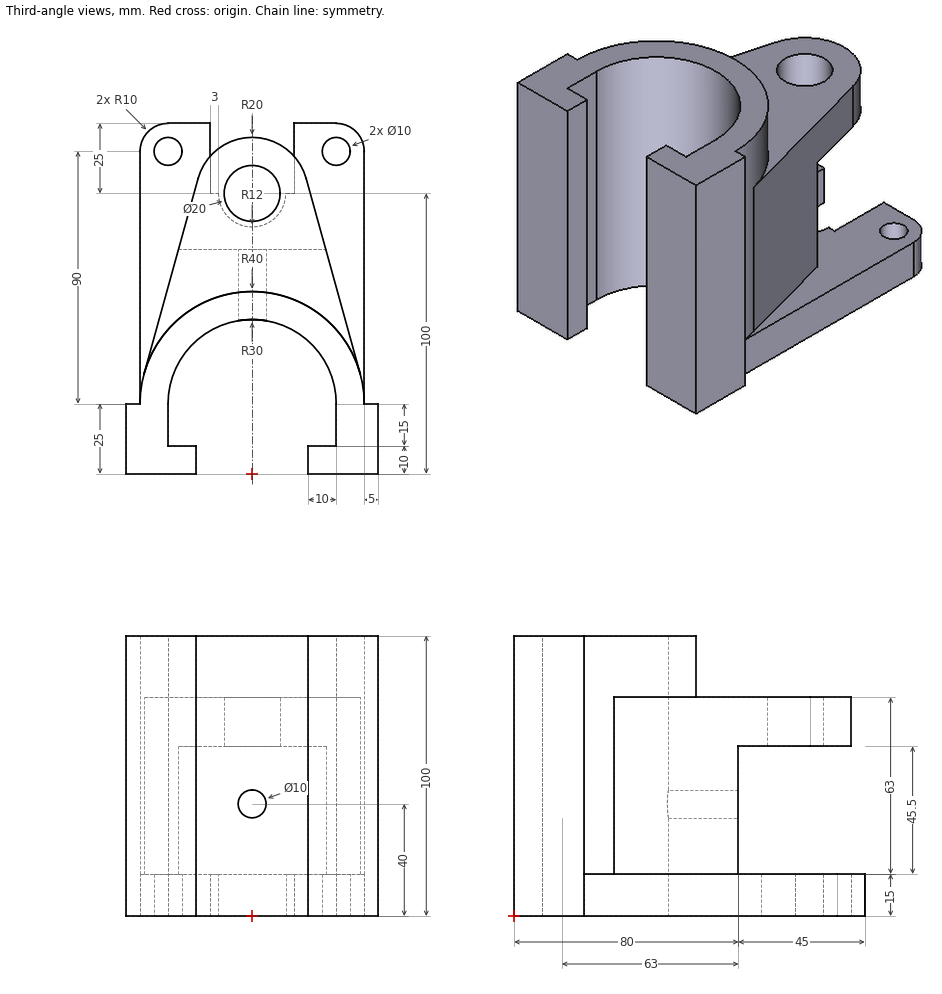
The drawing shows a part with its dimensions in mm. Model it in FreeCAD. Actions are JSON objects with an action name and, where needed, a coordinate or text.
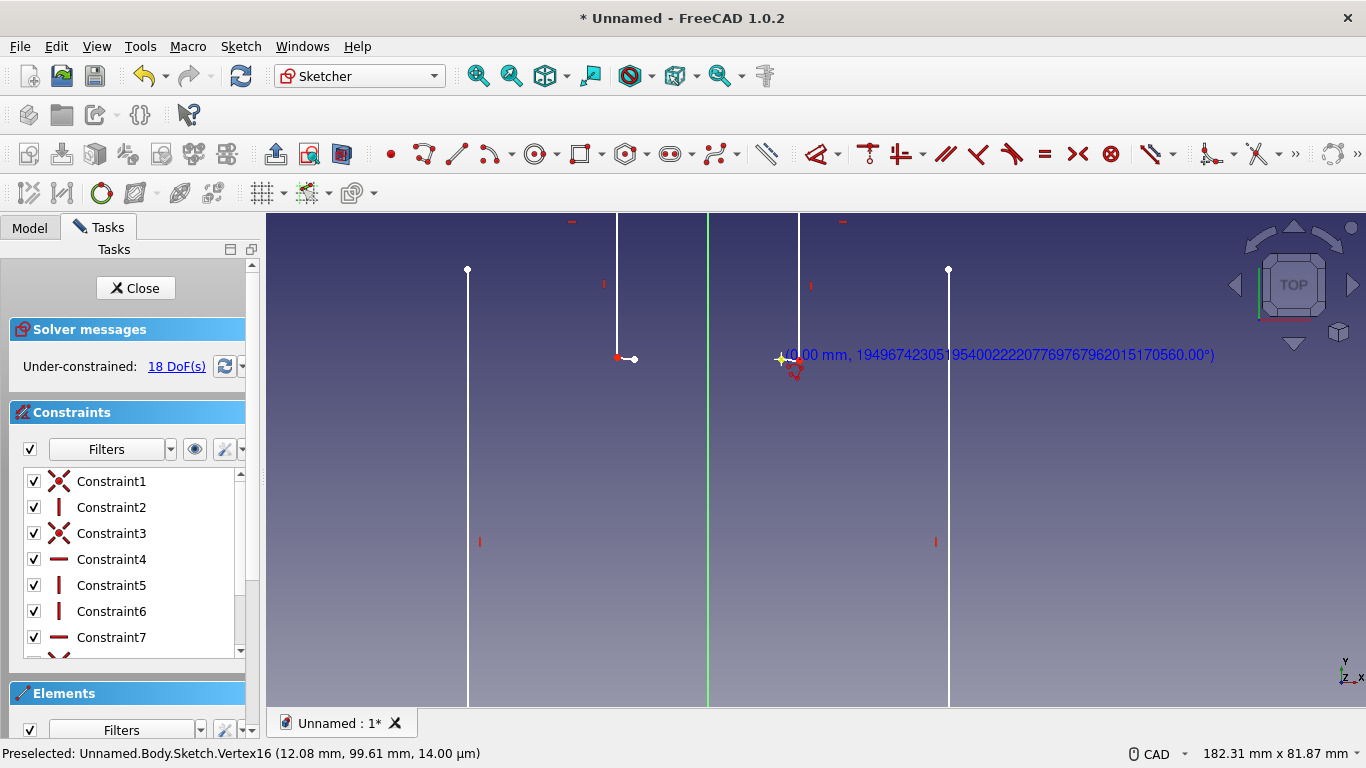
{"action": "key", "text": "g 3 a"}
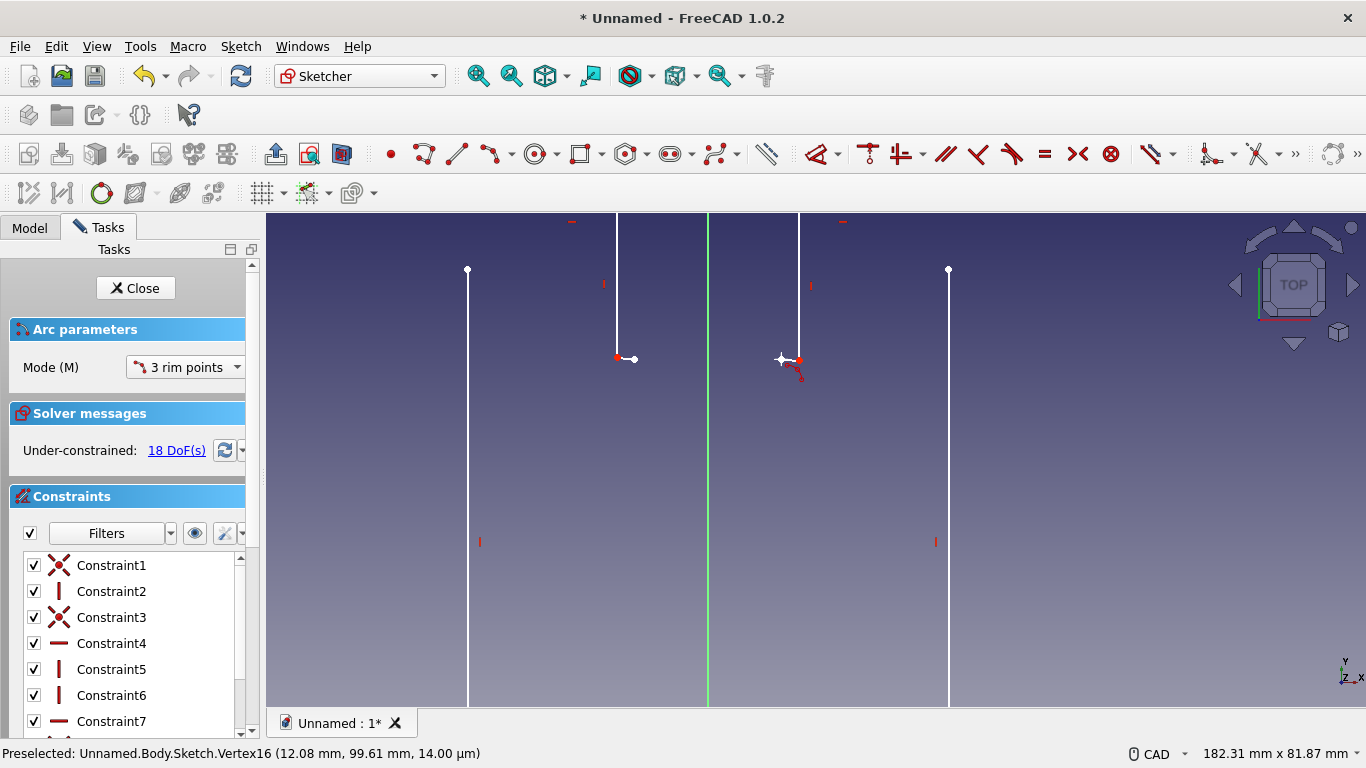
{"action": "scroll", "coordinate": [780, 359], "scroll_direction": "down", "scroll_amount": 4}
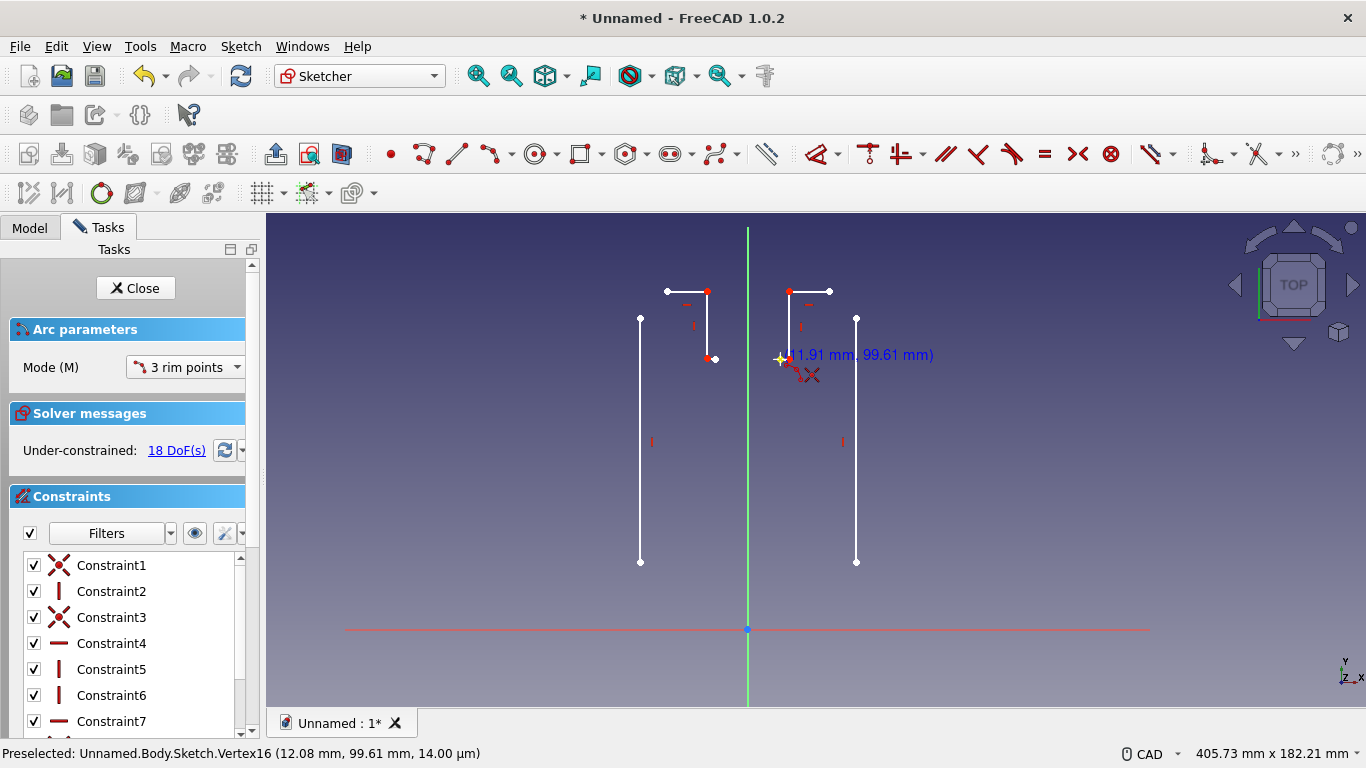
{"action": "left_click", "coordinate": [667, 292]}
{"action": "left_click", "coordinate": [640, 319]}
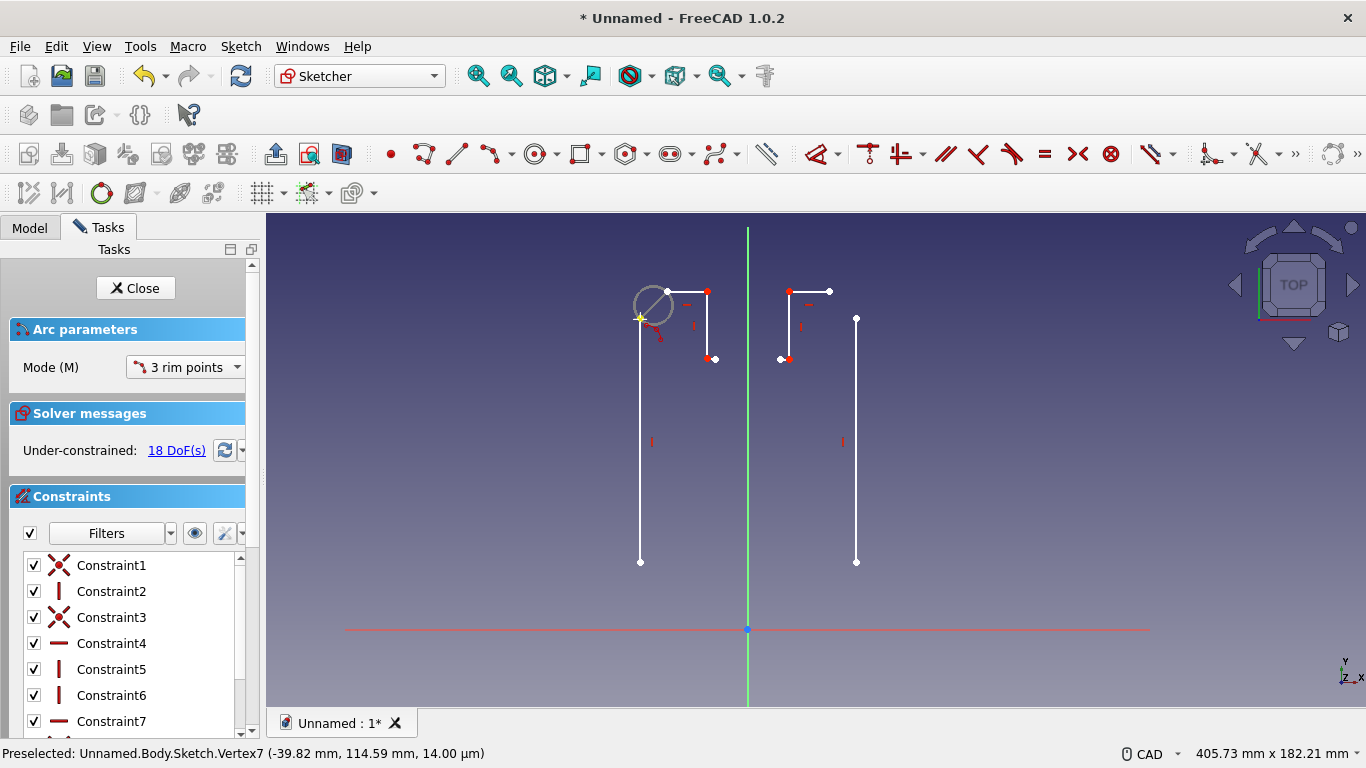
{"action": "scroll", "coordinate": [647, 299], "scroll_direction": "up", "scroll_amount": 4}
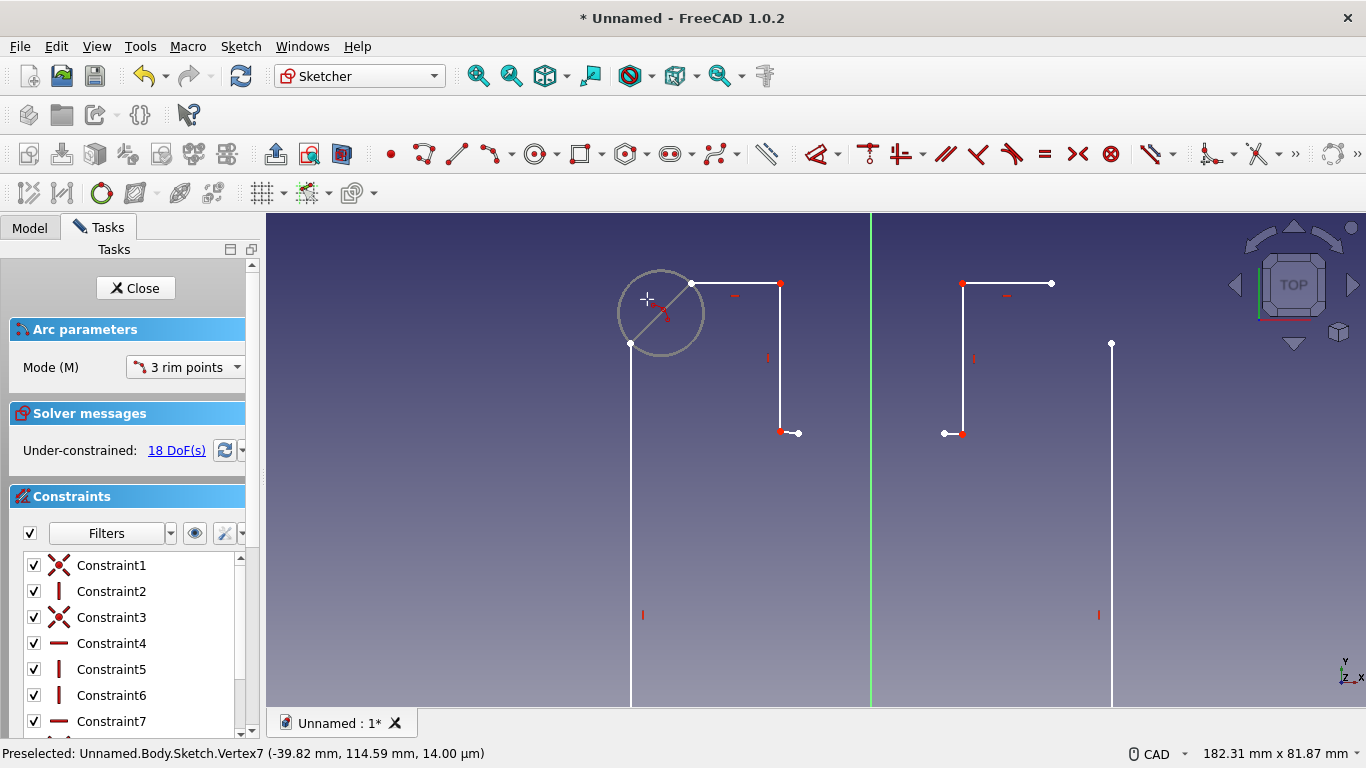
{"action": "left_click", "coordinate": [648, 298]}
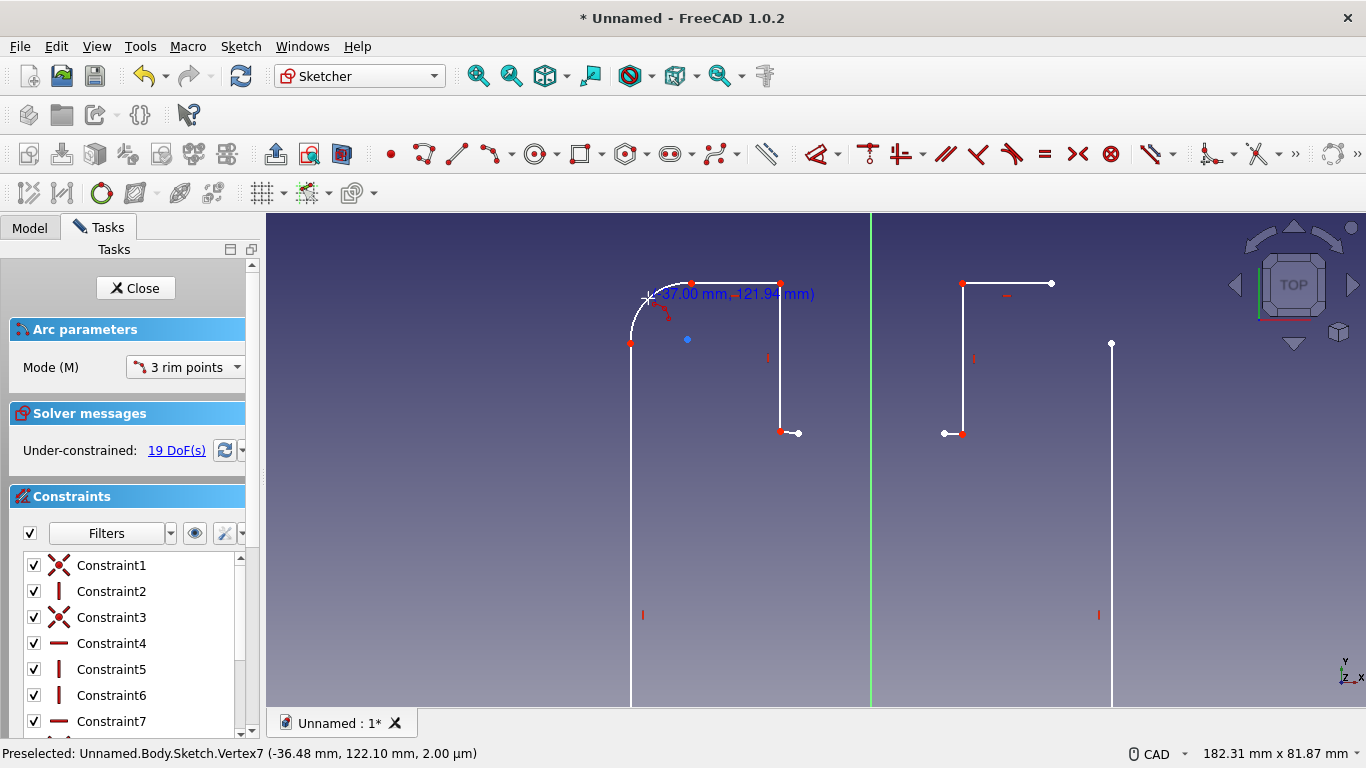
{"action": "scroll", "coordinate": [647, 299], "scroll_direction": "down", "scroll_amount": 4}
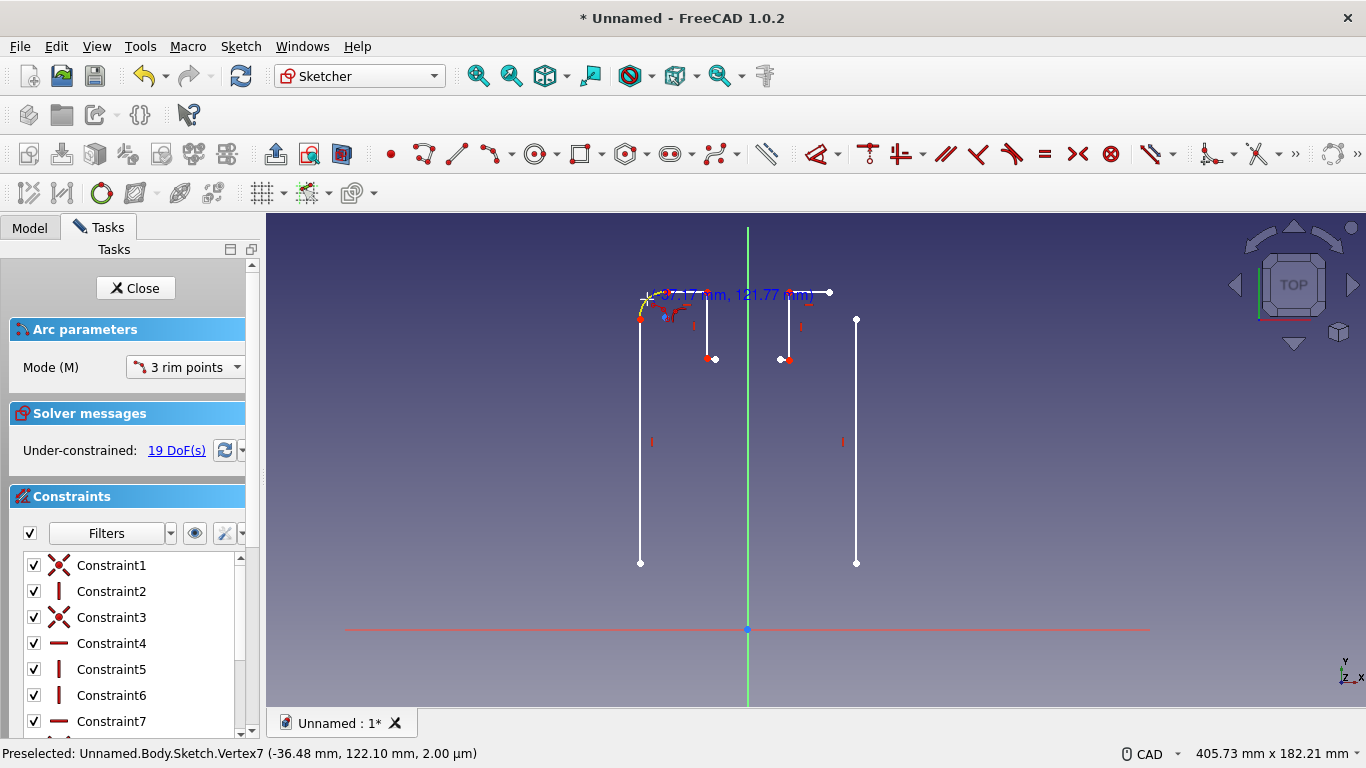
{"action": "left_click", "coordinate": [640, 563]}
{"action": "left_click", "coordinate": [856, 563]}
{"action": "left_click", "coordinate": [781, 459]}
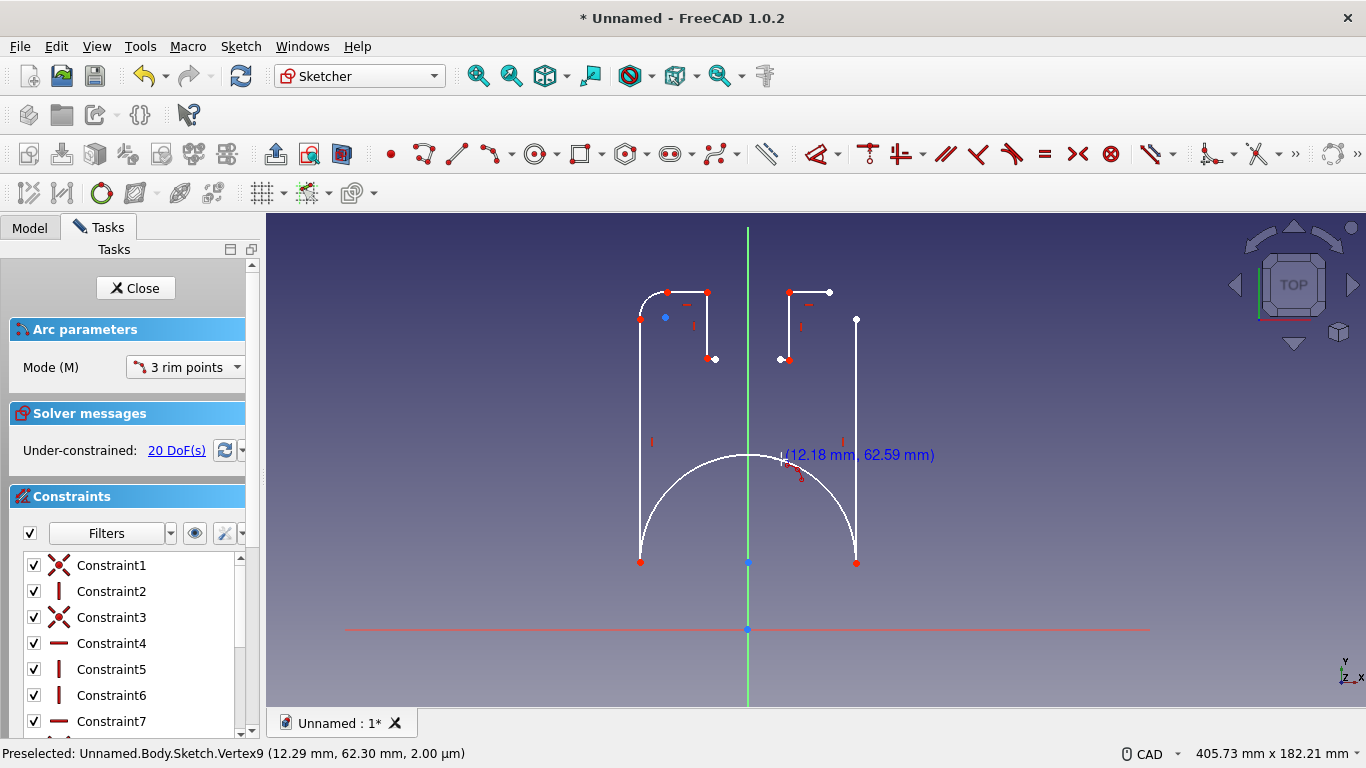
{"action": "left_click", "coordinate": [856, 319]}
{"action": "left_click", "coordinate": [829, 292]}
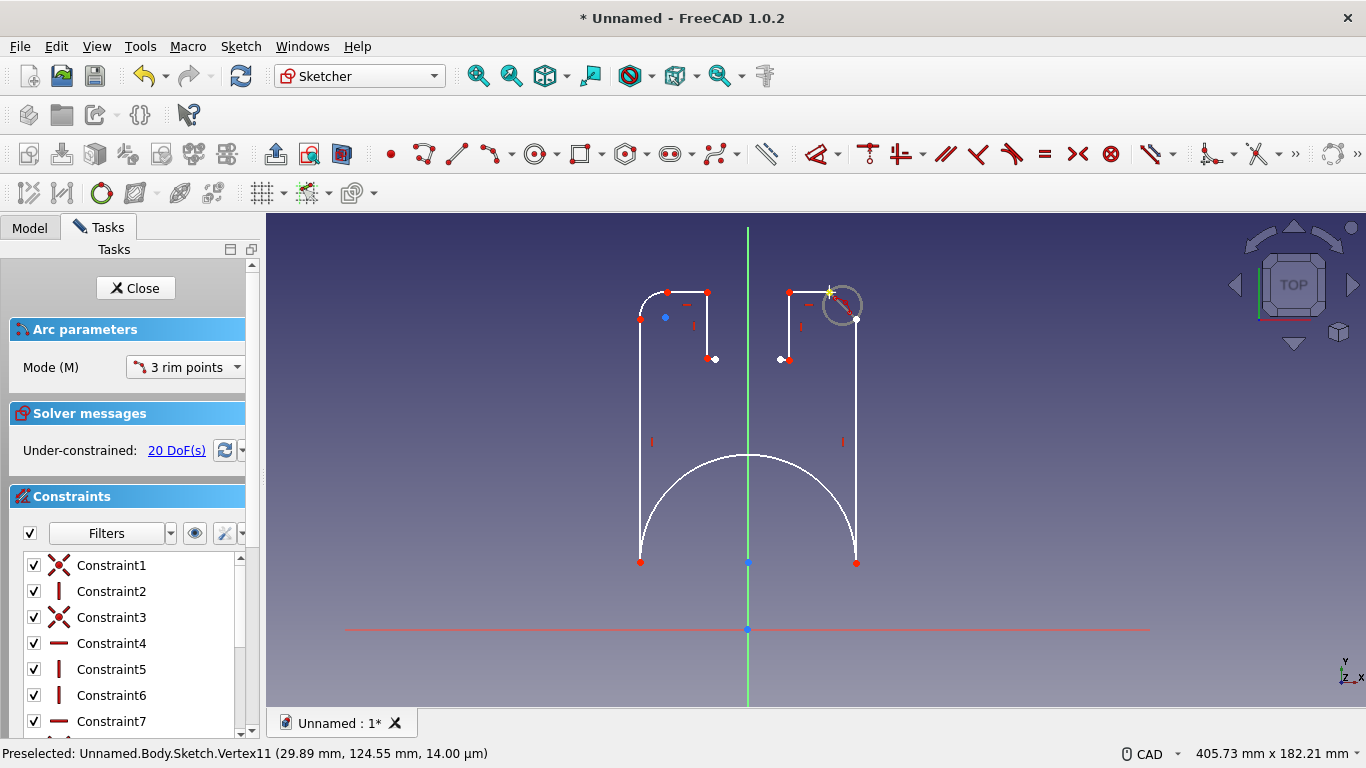
{"action": "scroll", "coordinate": [848, 299], "scroll_direction": "up", "scroll_amount": 4}